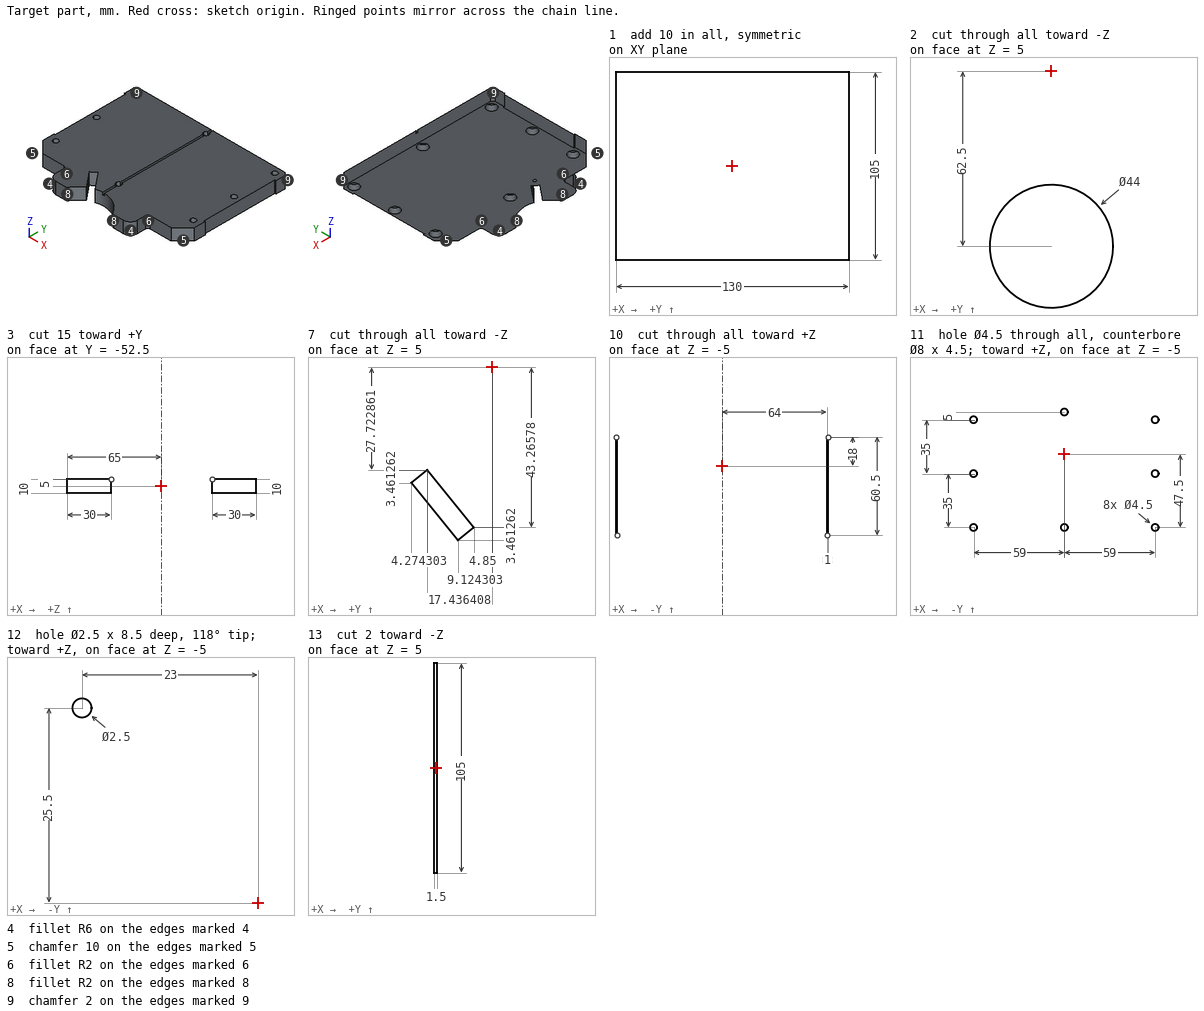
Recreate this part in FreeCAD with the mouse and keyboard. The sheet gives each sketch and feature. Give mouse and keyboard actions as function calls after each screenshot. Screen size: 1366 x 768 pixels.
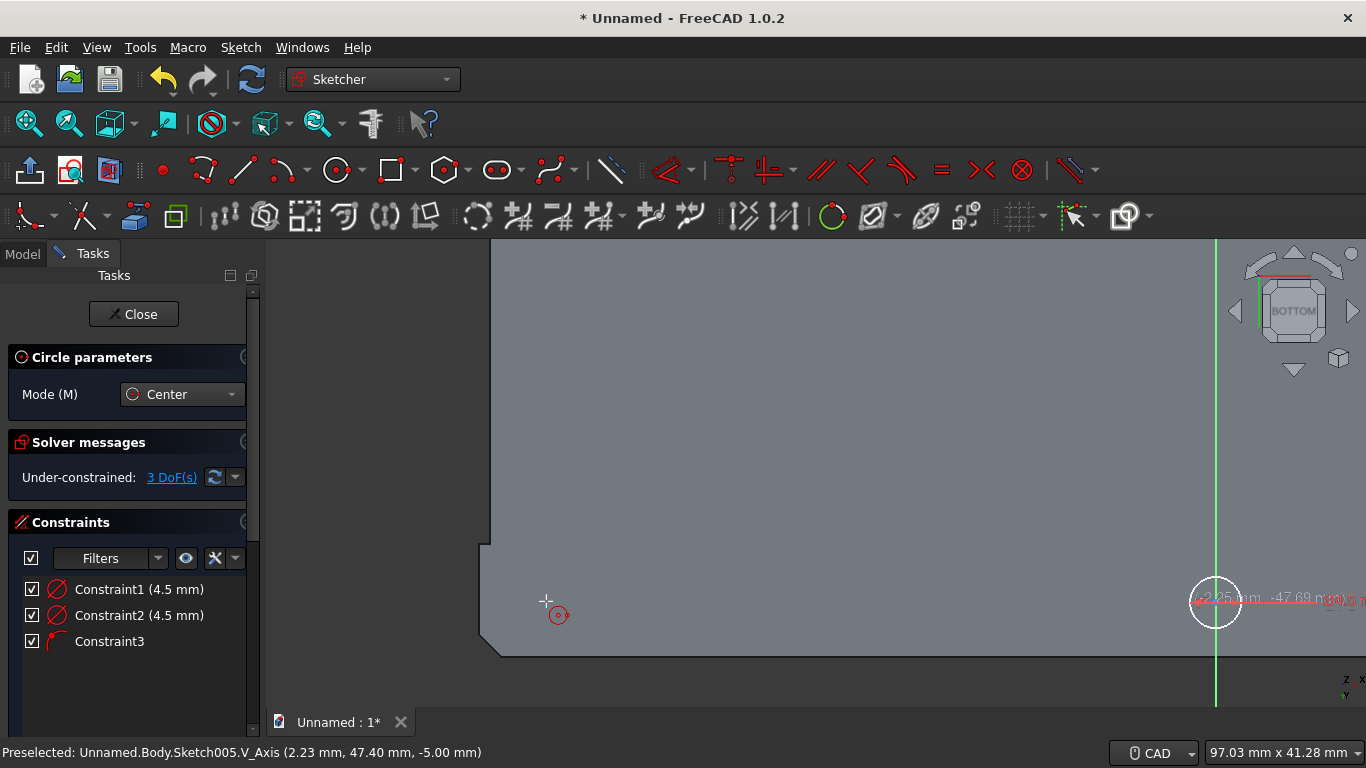
scroll(546, 601, down, 6)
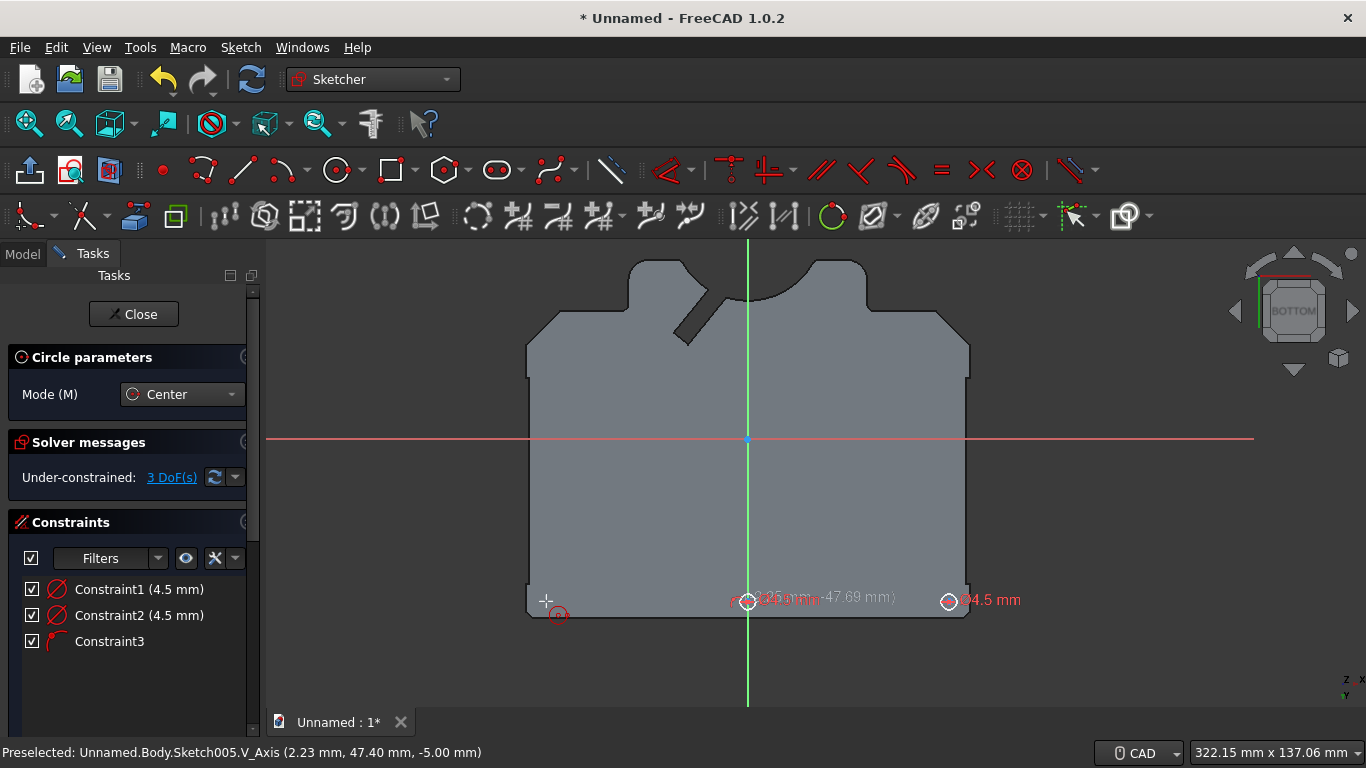
click(546, 601)
move(552, 596)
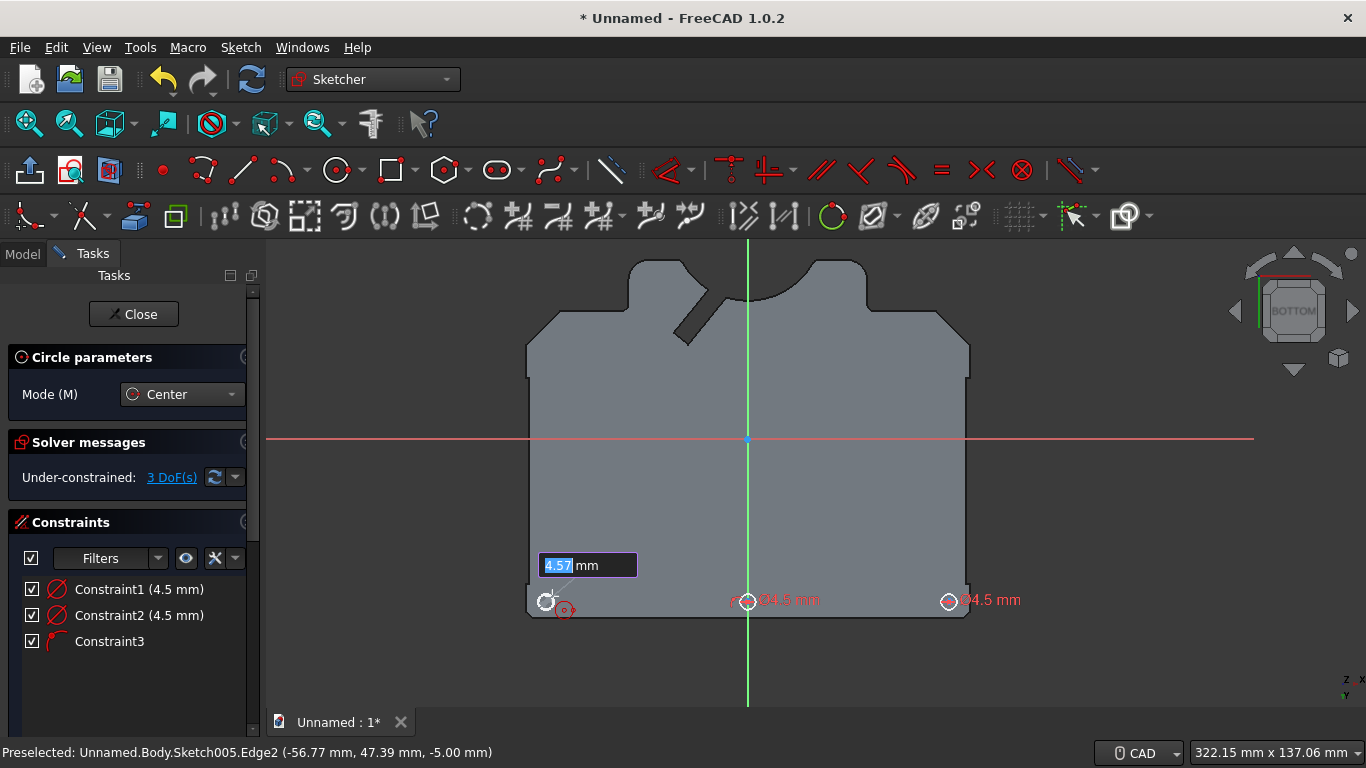
text(4.5)
key(Return)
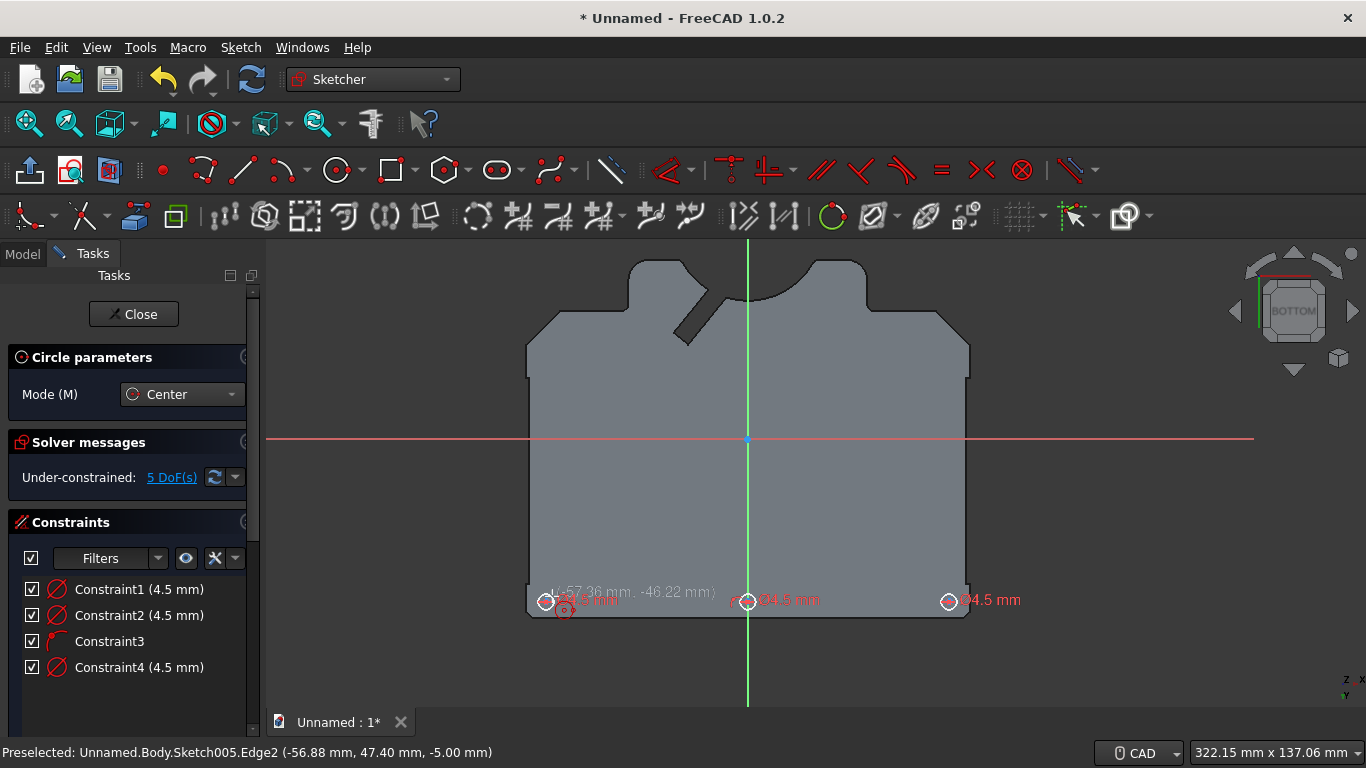
scroll(546, 482, up, 6)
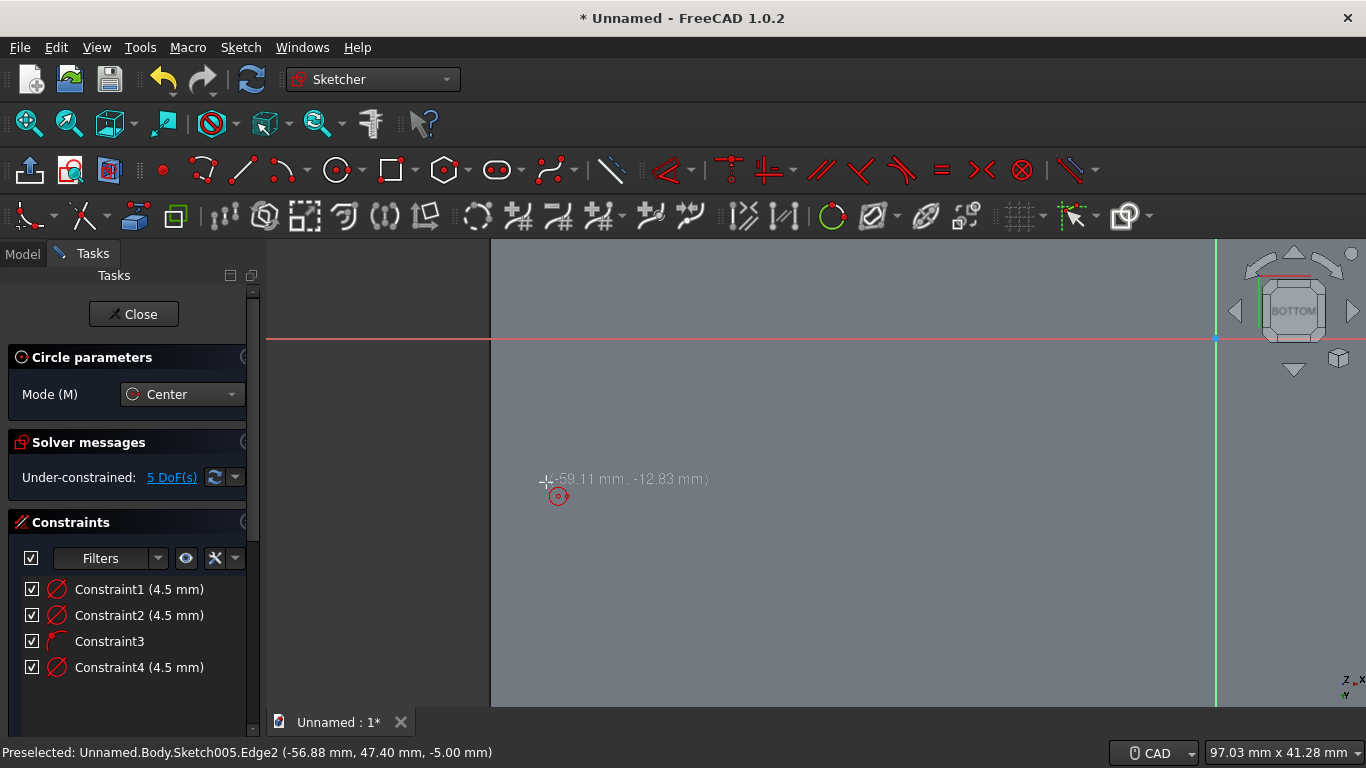
scroll(546, 482, down, 6)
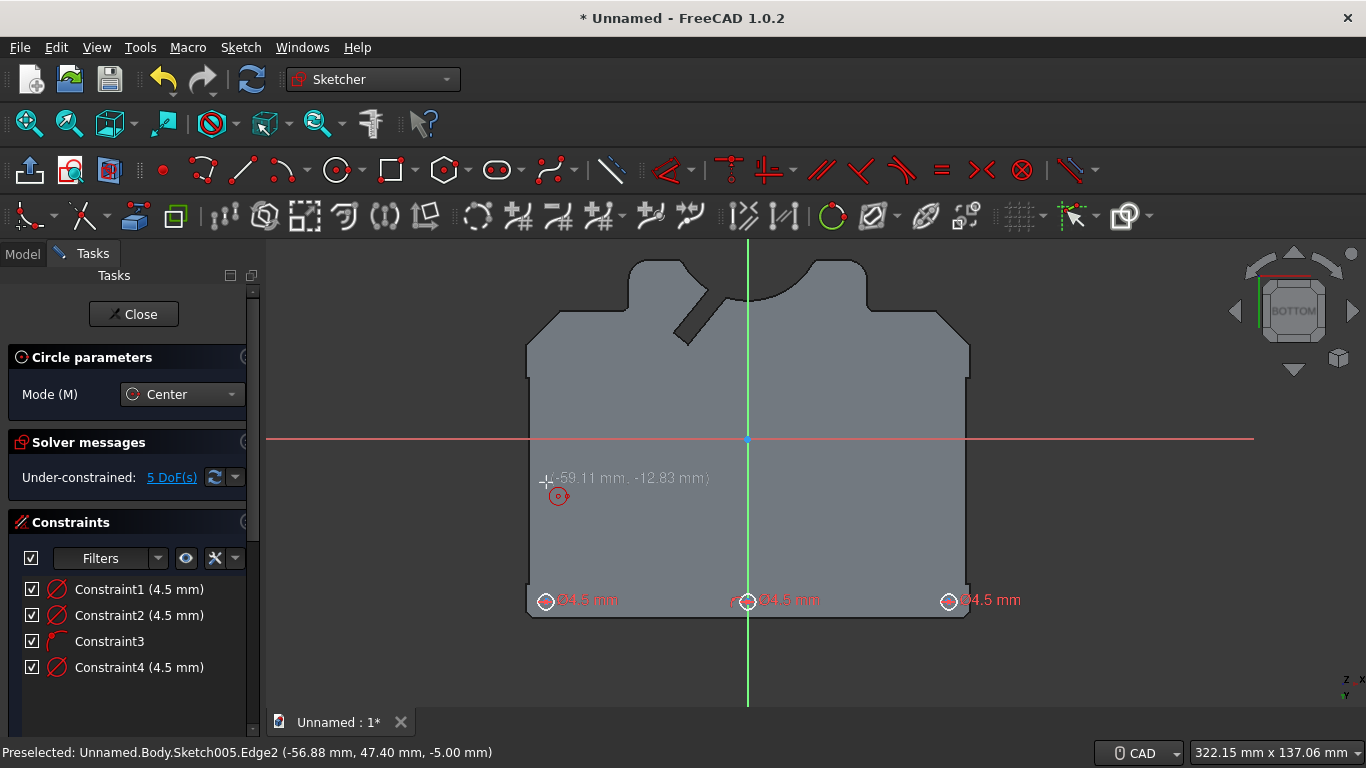
click(546, 482)
move(552, 476)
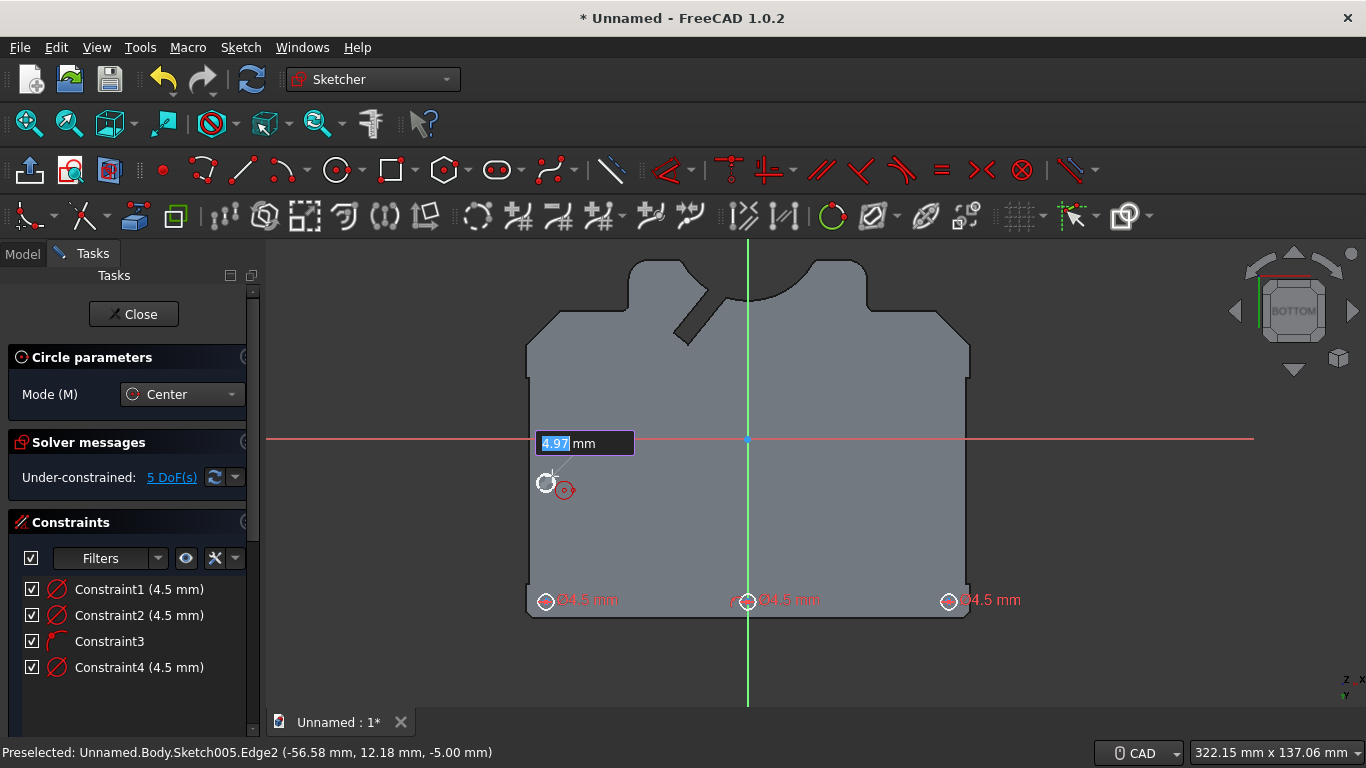
text(4.5)
key(Return)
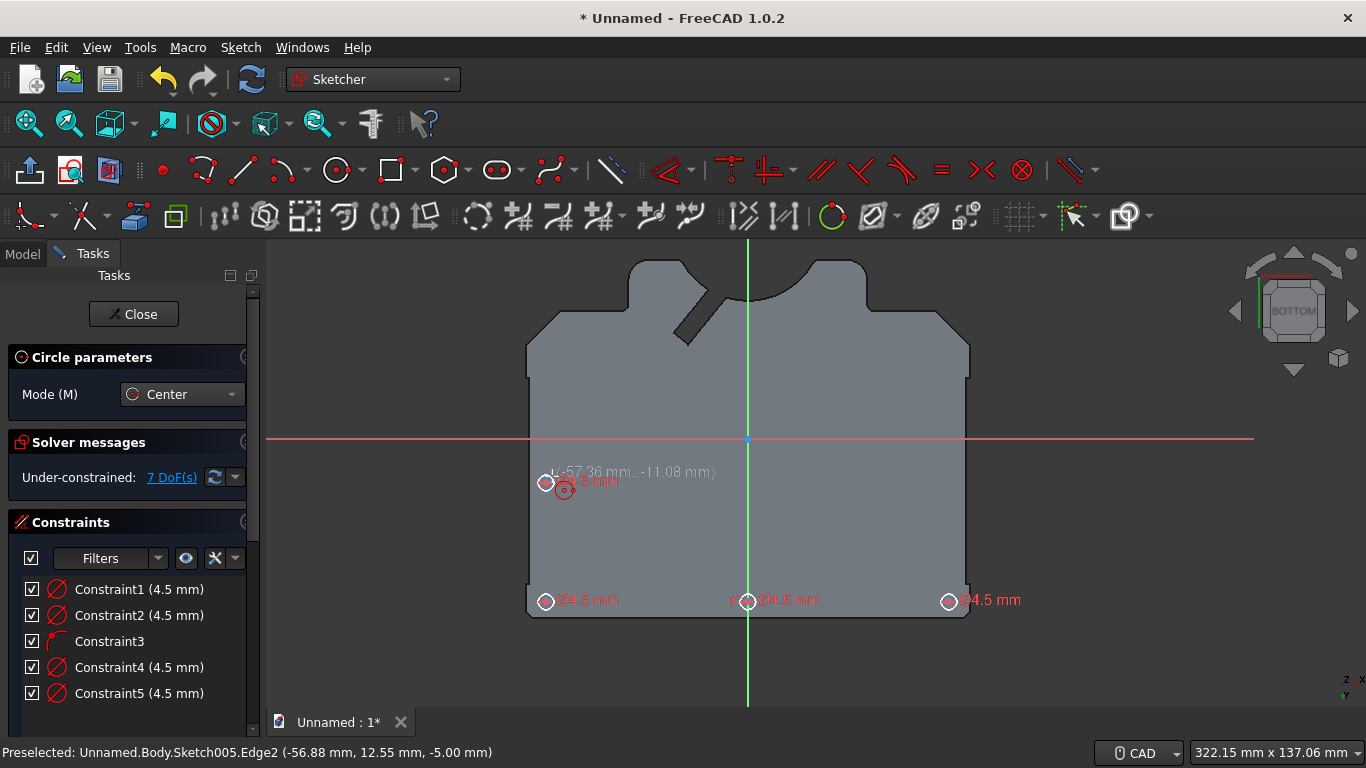
scroll(546, 362, up, 6)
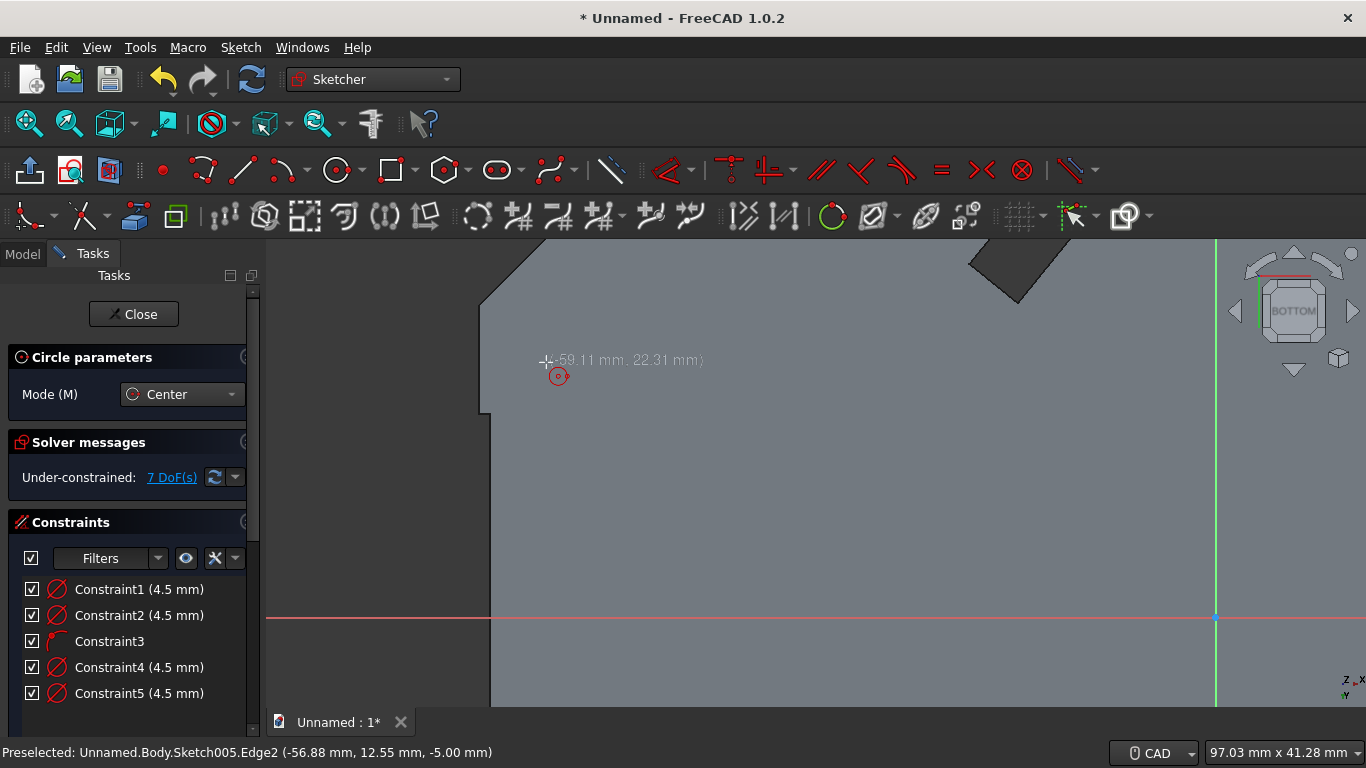
scroll(546, 362, down, 6)